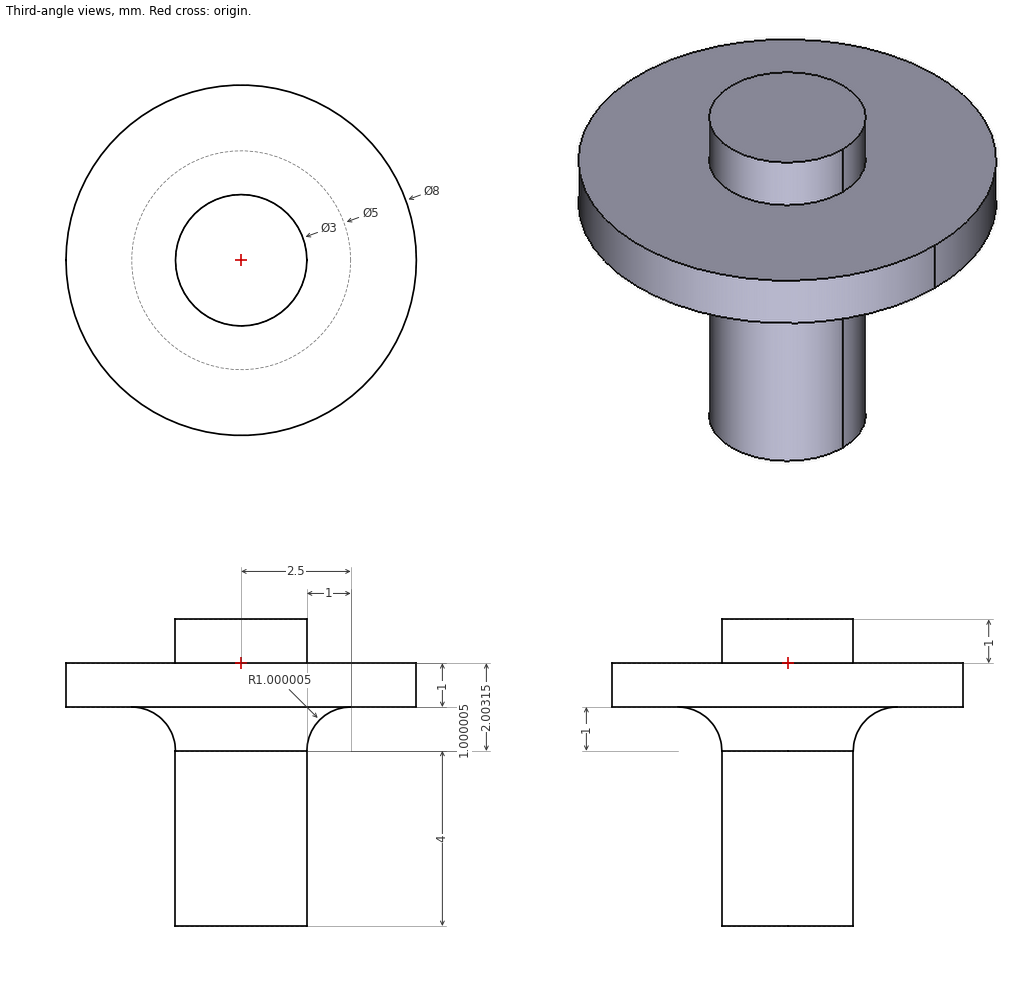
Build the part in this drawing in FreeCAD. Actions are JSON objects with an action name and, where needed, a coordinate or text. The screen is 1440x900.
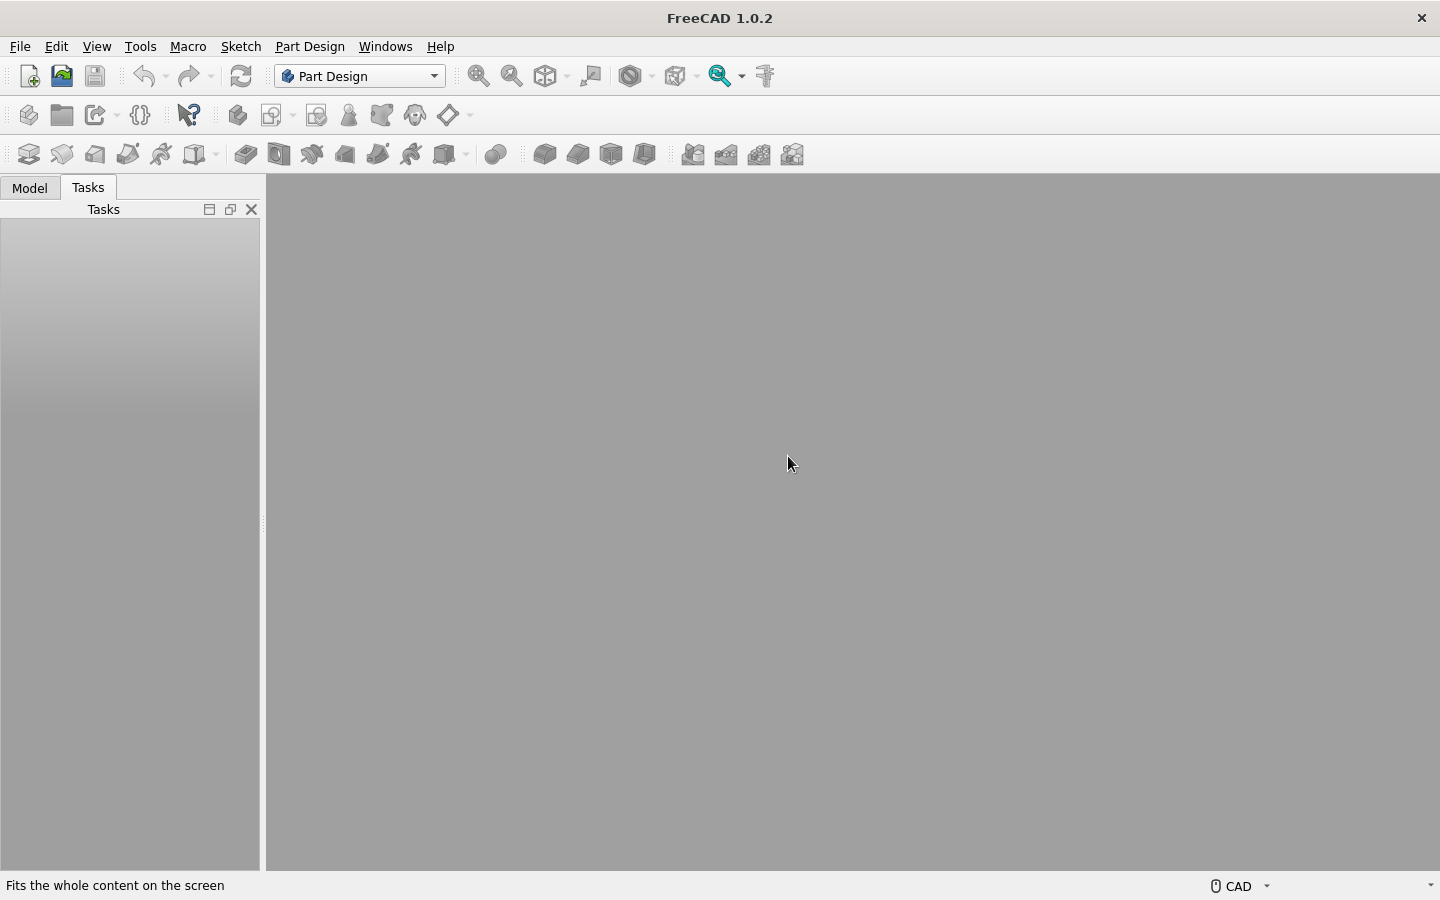
{"action": "left_click", "coordinate": [29, 76]}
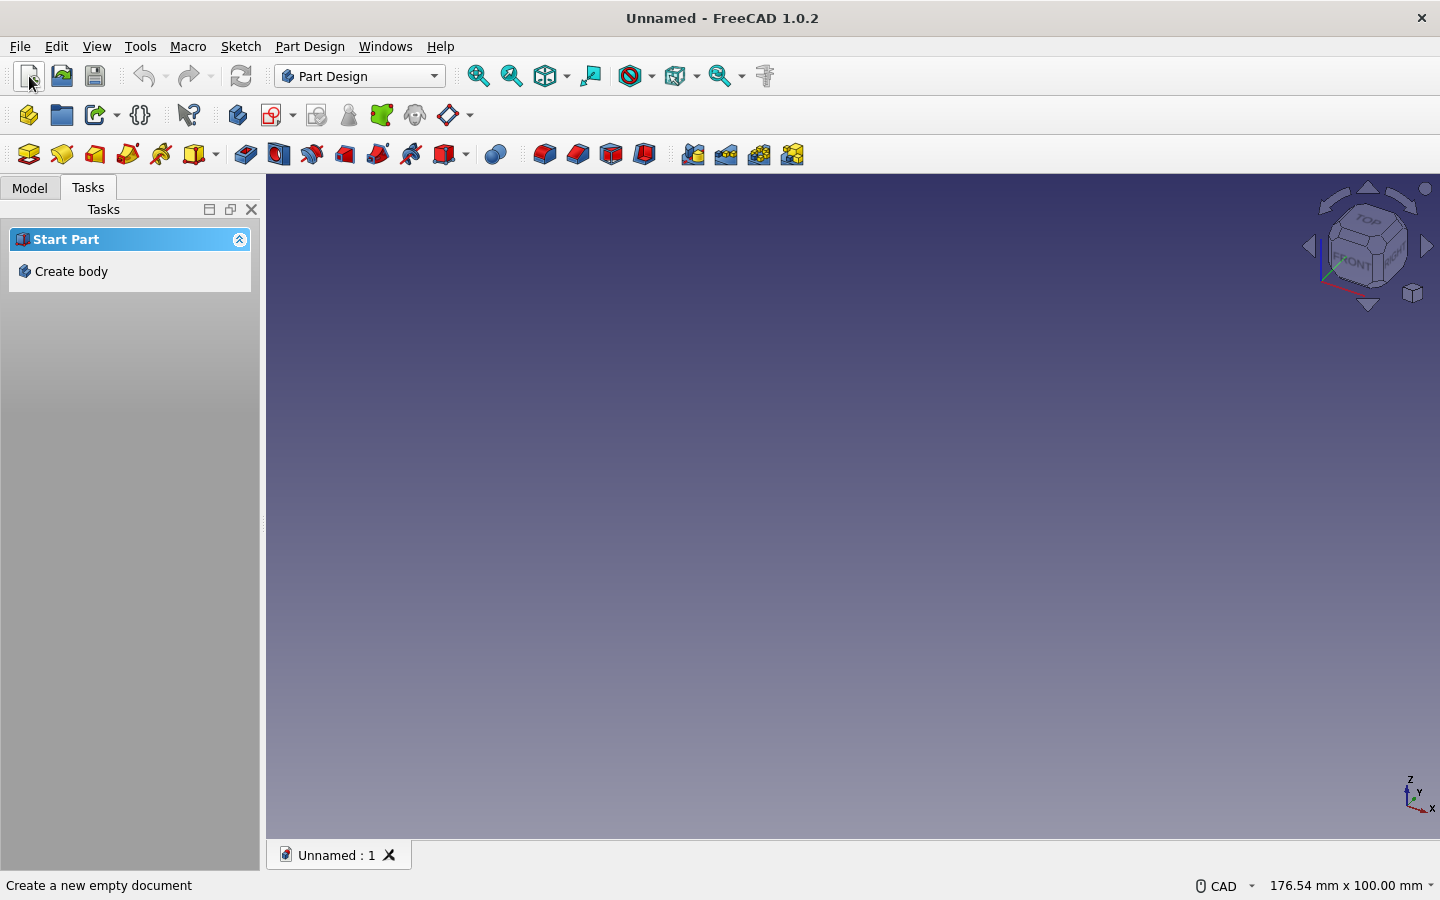
{"action": "left_click", "coordinate": [270, 116]}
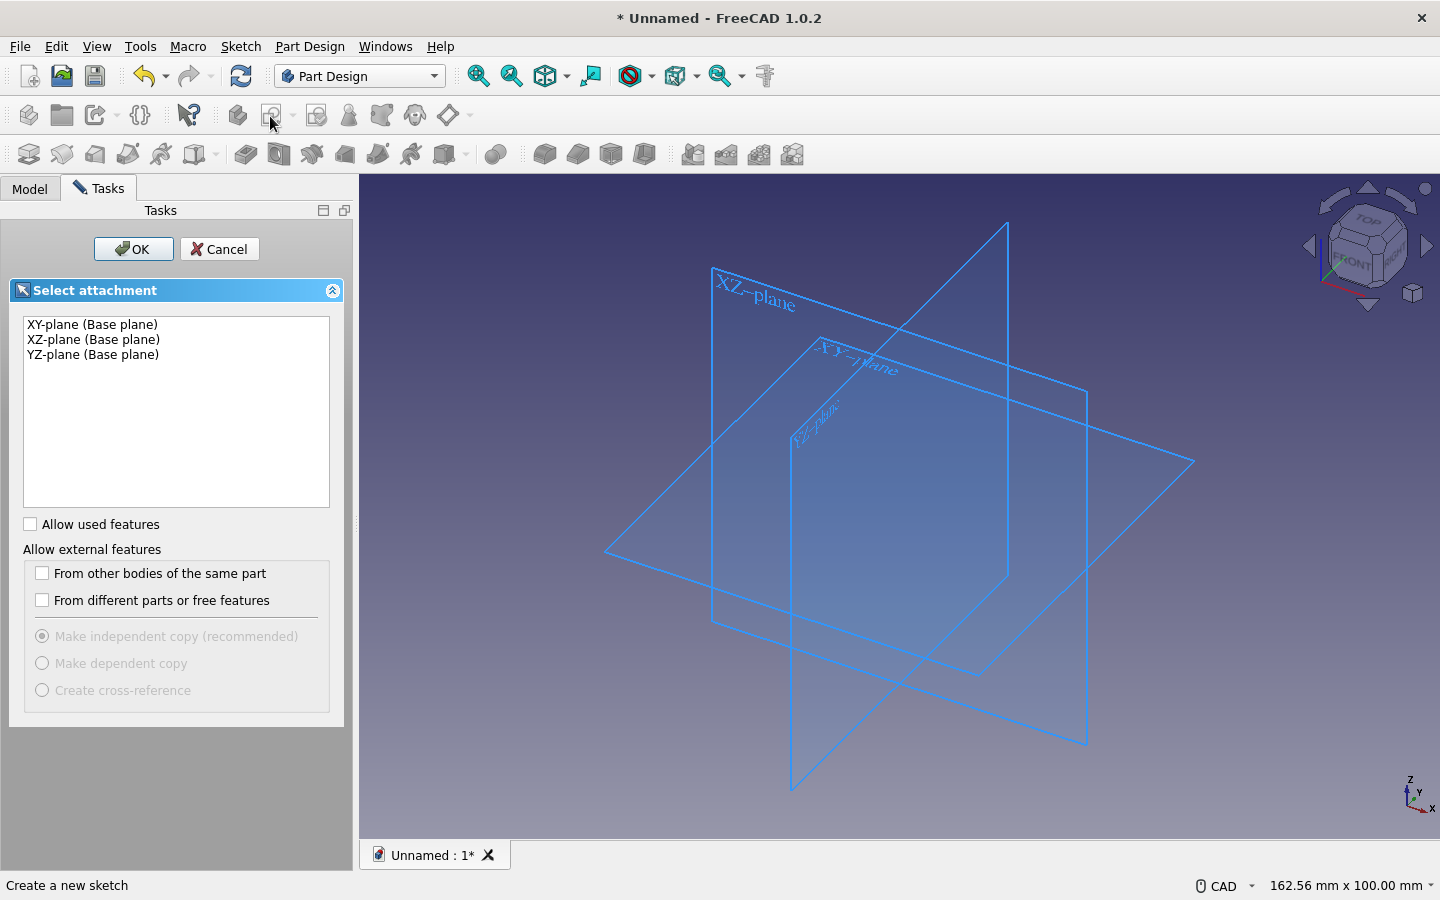
{"action": "left_click", "coordinate": [84, 324]}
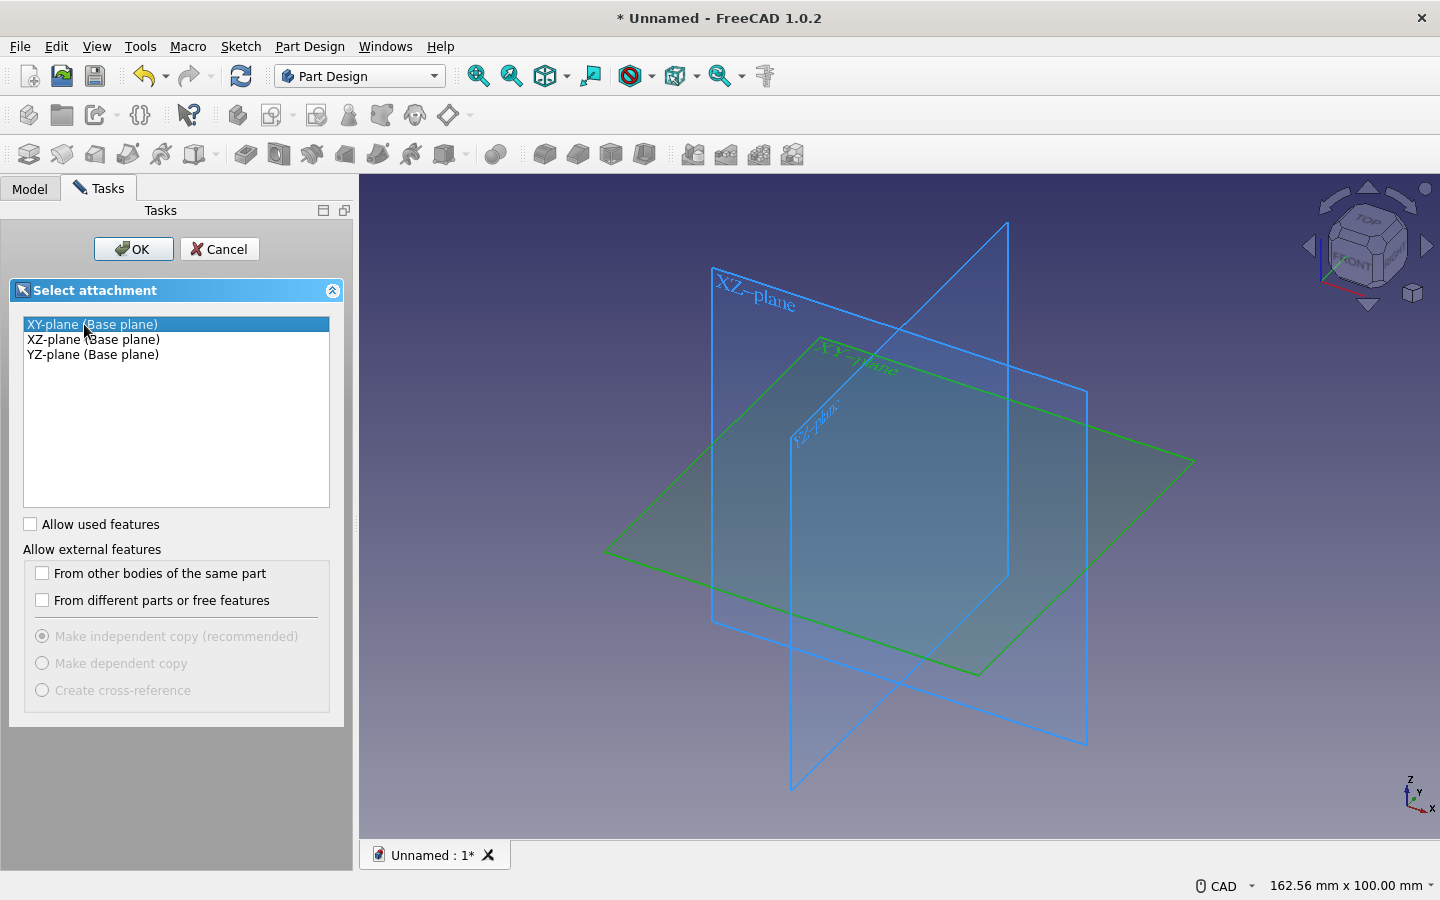
{"action": "left_click", "coordinate": [134, 249]}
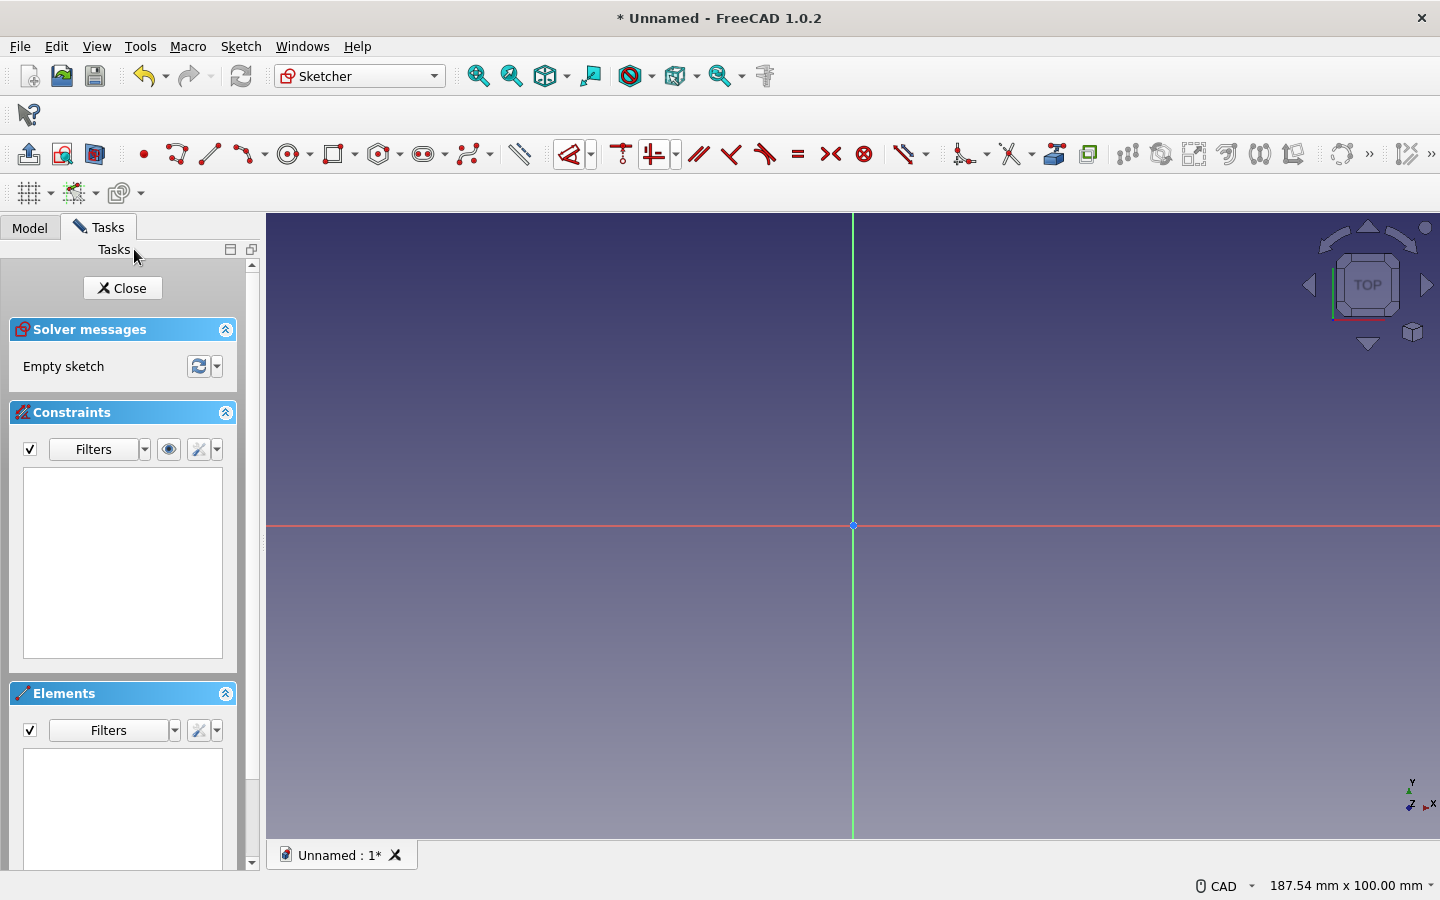
{"action": "scroll", "coordinate": [857, 526], "scroll_direction": "up", "scroll_amount": 15}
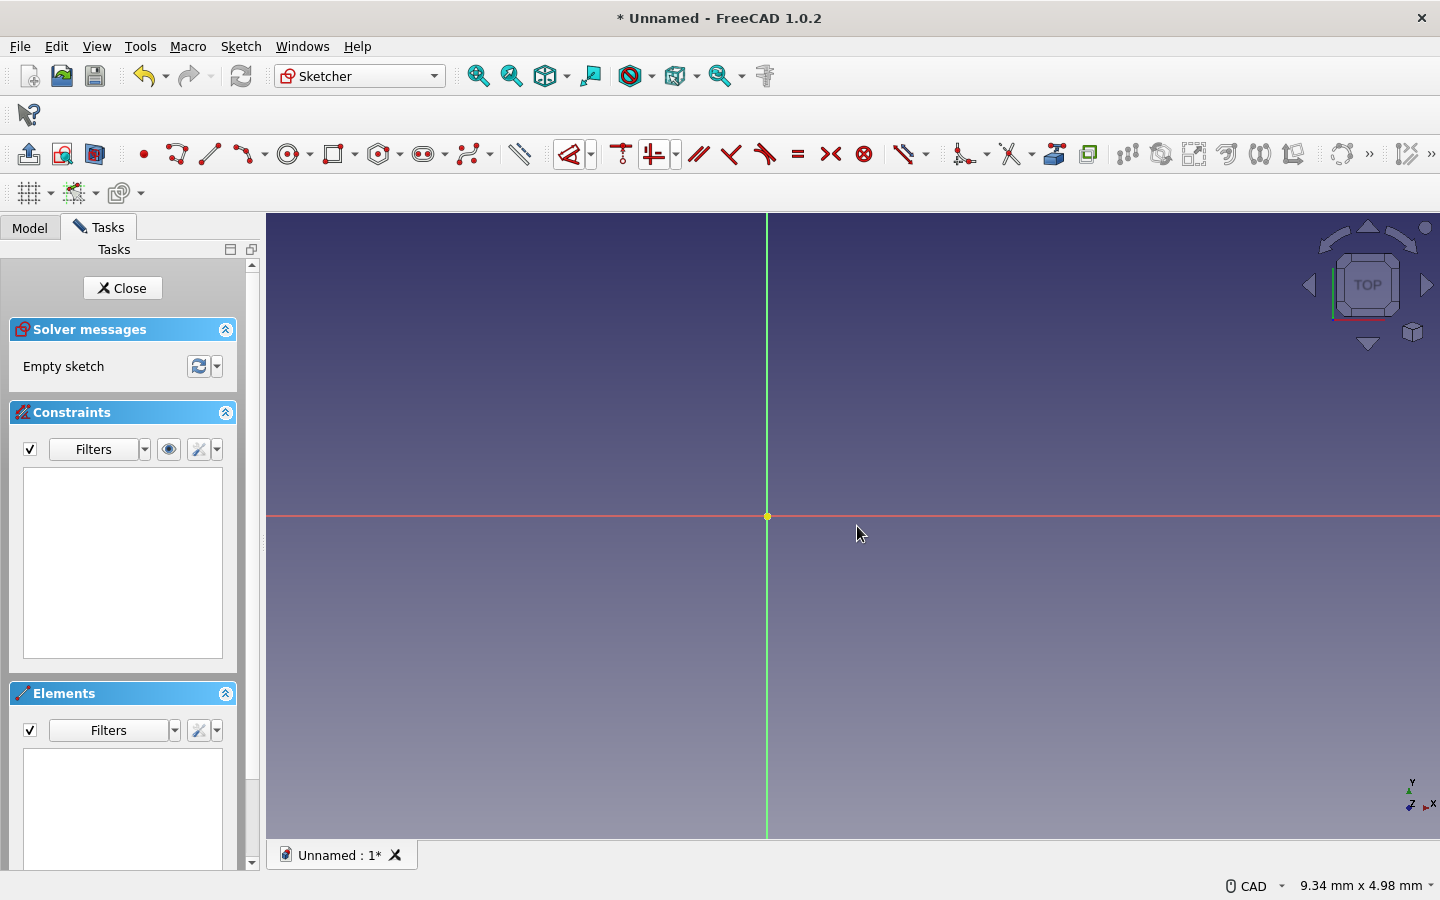
{"action": "left_click", "coordinate": [288, 154]}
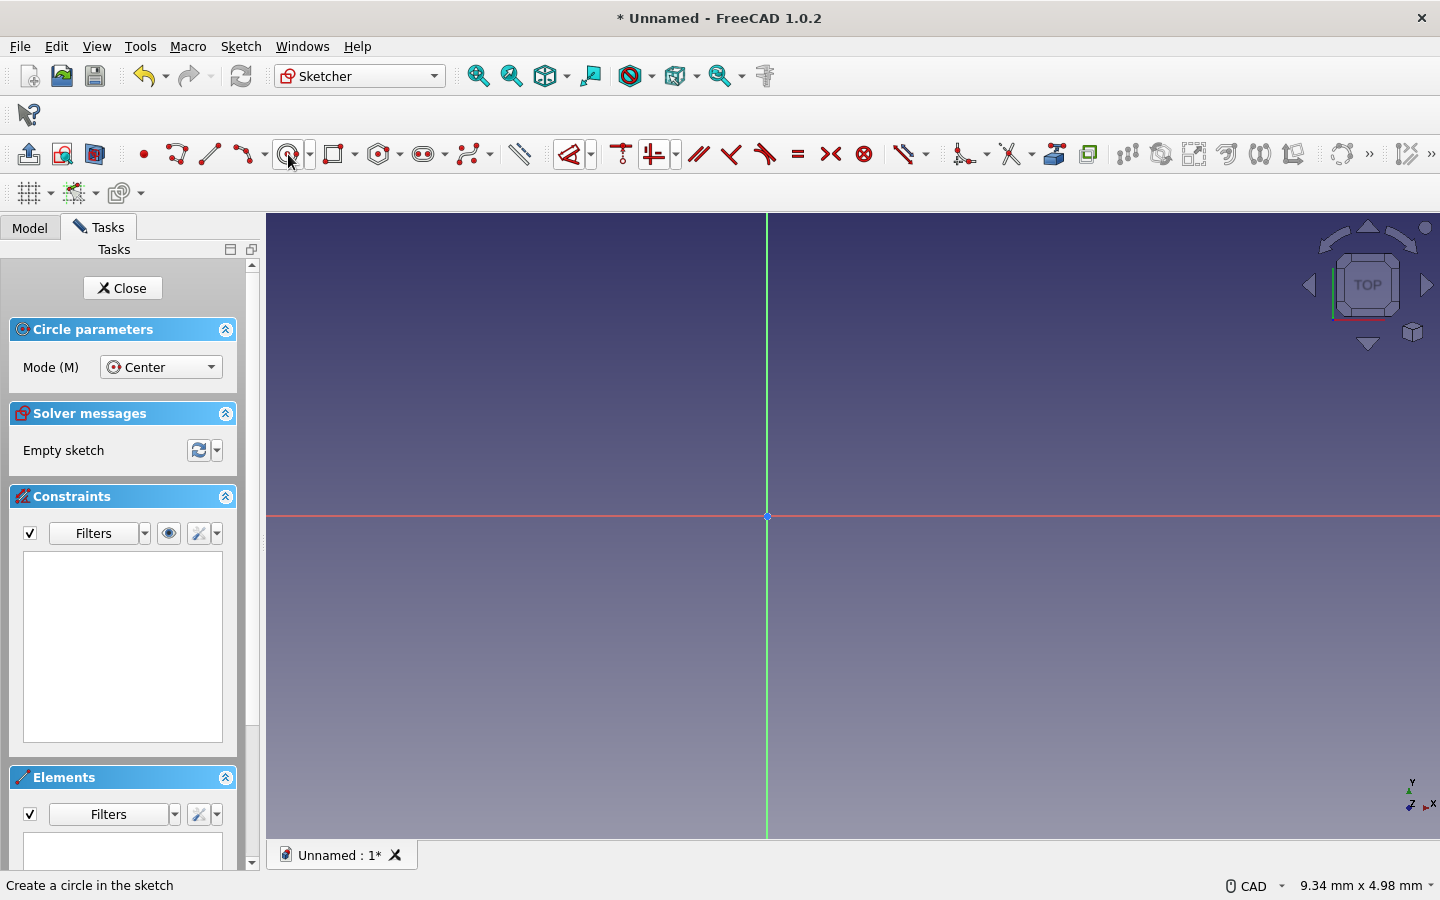
{"action": "left_click", "coordinate": [767, 516]}
{"action": "left_click", "coordinate": [900, 383]}
{"action": "key", "text": "Escape"}